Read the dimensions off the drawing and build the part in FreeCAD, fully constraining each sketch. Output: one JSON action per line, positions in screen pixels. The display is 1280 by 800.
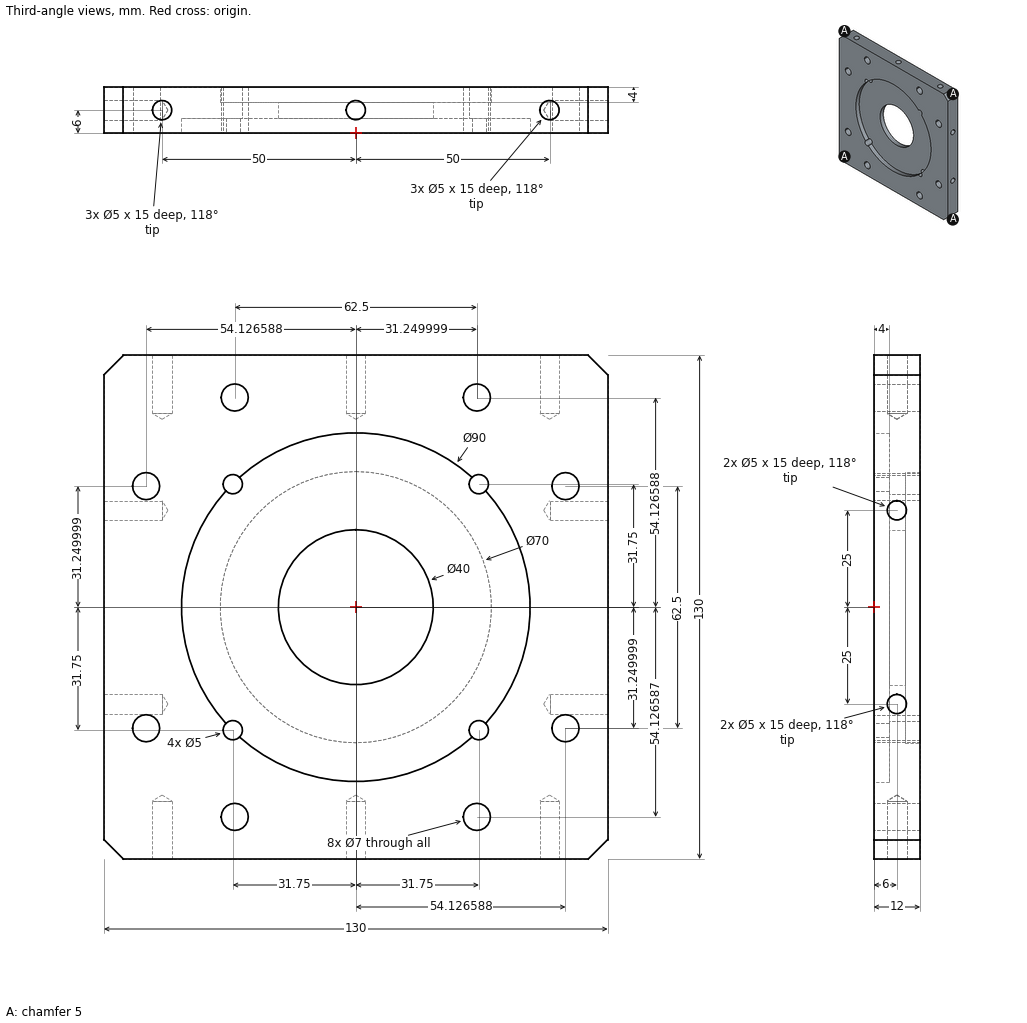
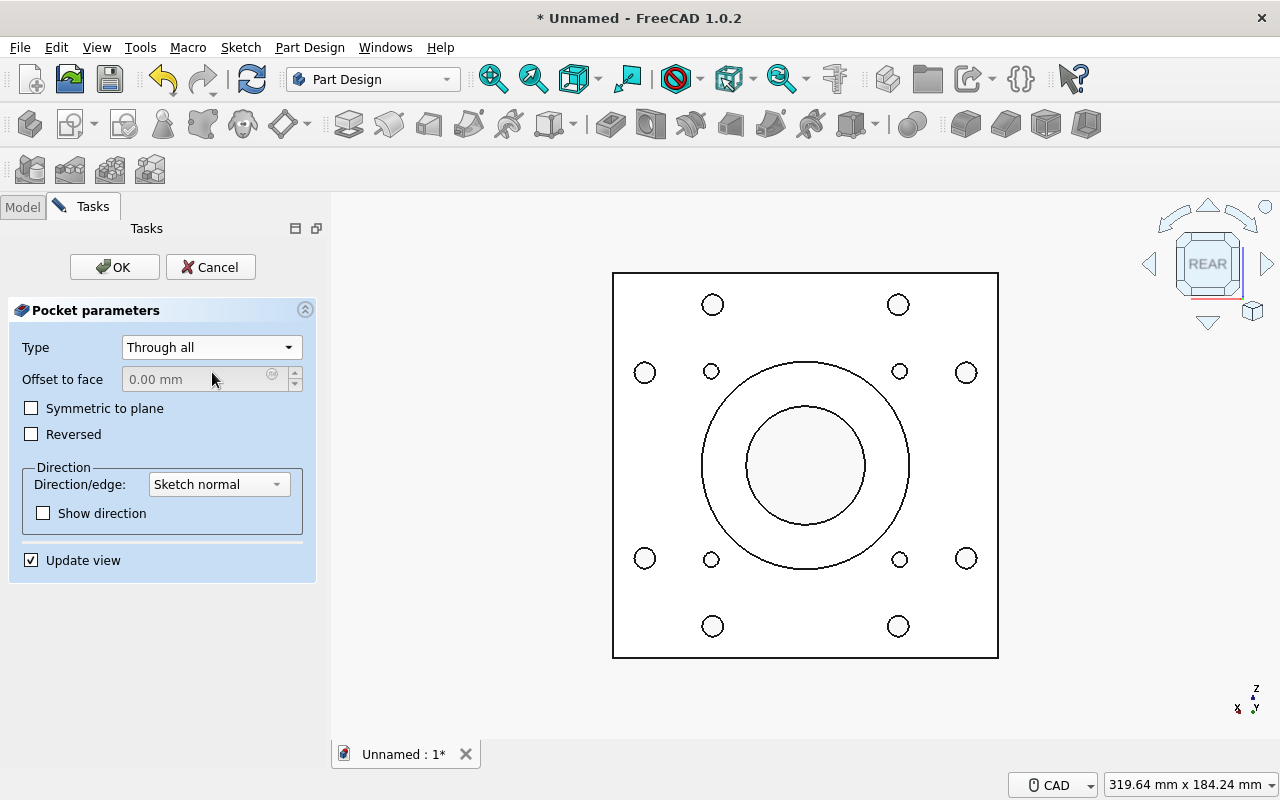
{"action": "left_click", "coordinate": [115, 267]}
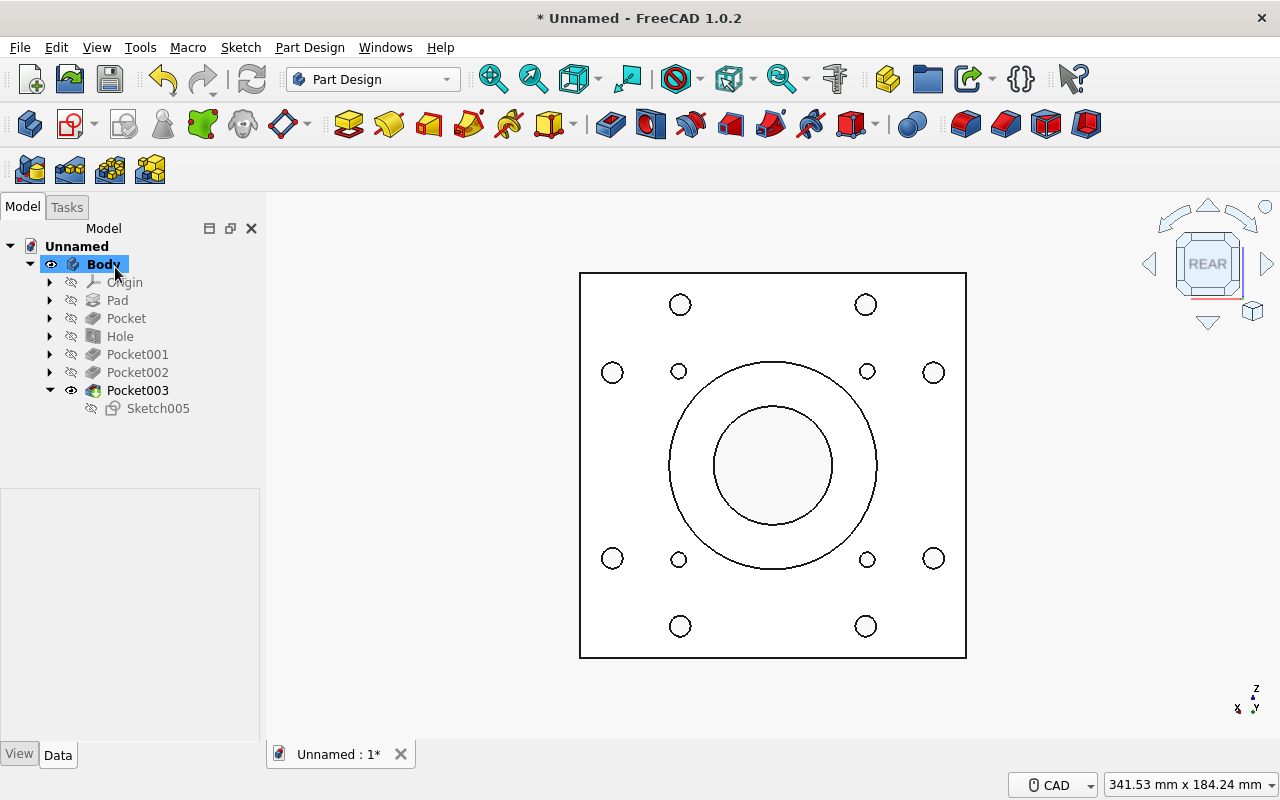
{"action": "key", "text": "6"}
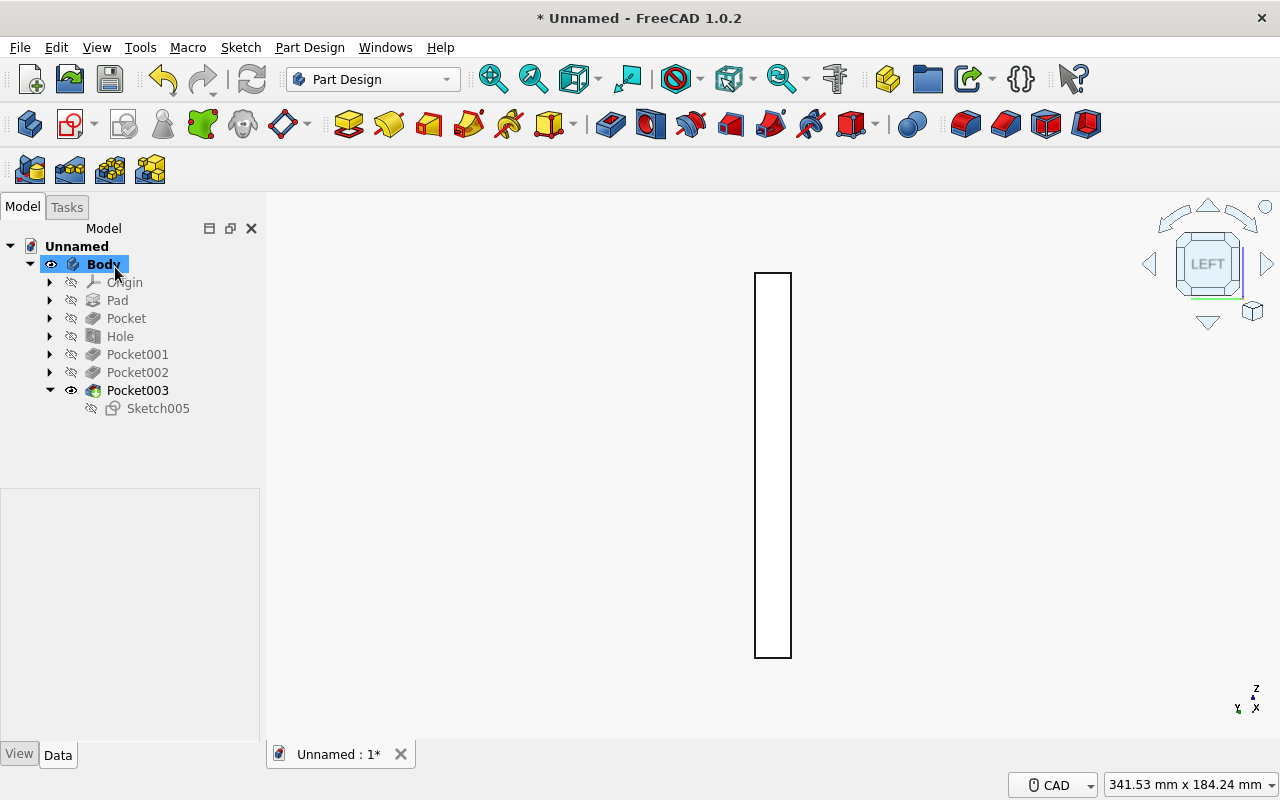
{"action": "left_click", "coordinate": [773, 299]}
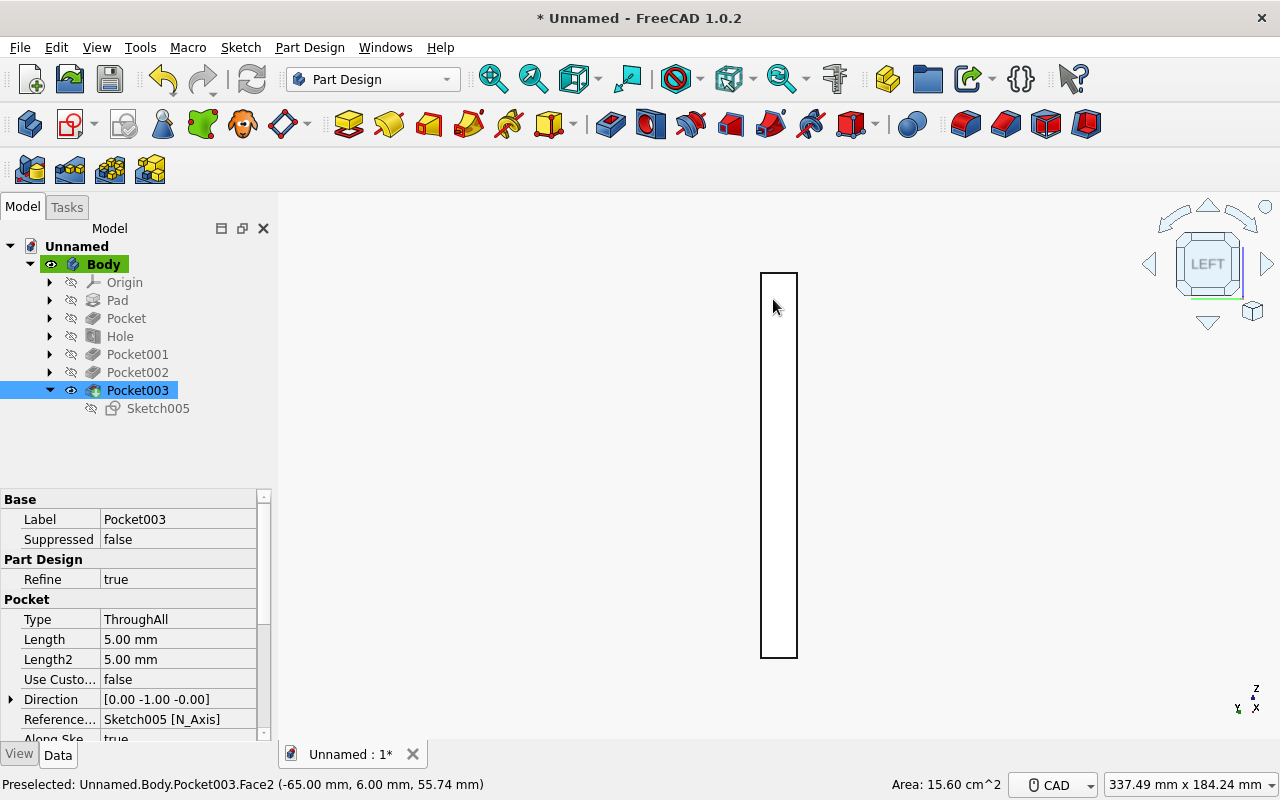
{"action": "left_click", "coordinate": [70, 124]}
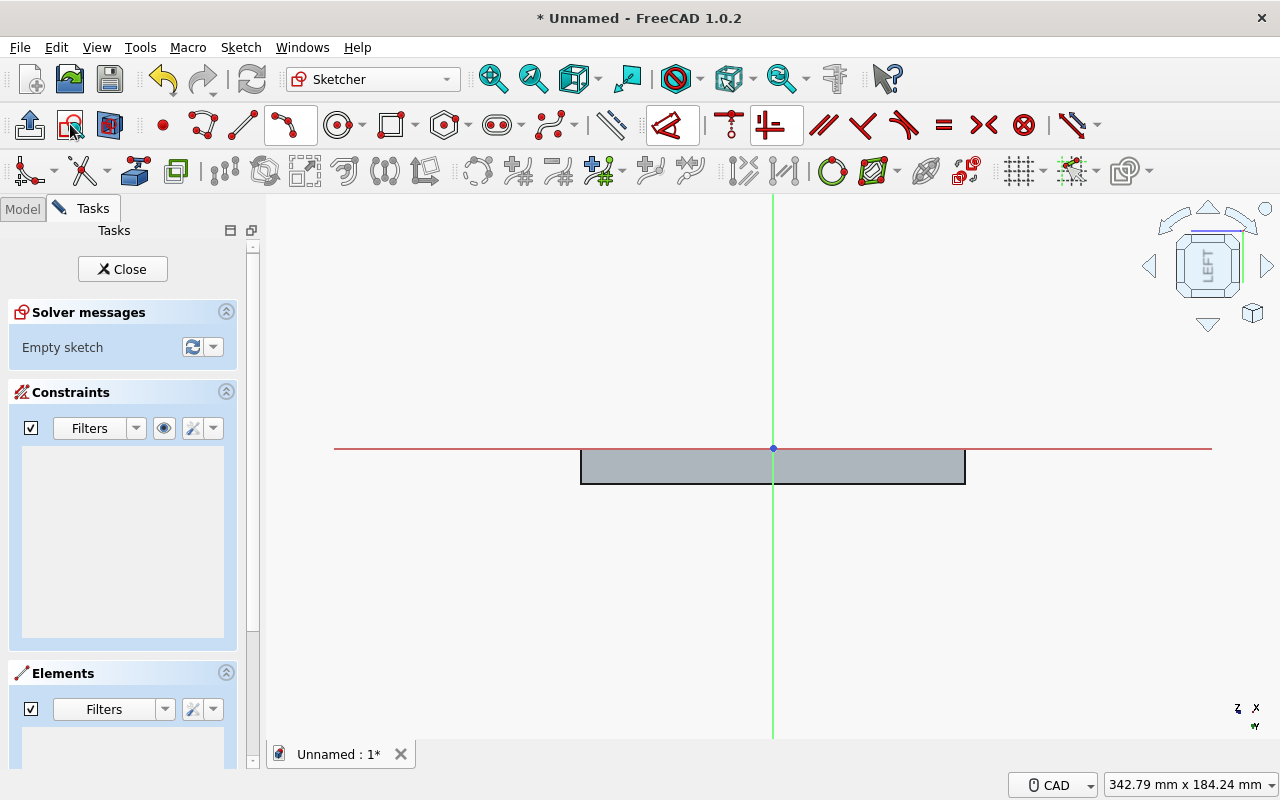
{"action": "scroll", "coordinate": [803, 459], "scroll_direction": "up", "scroll_amount": 6}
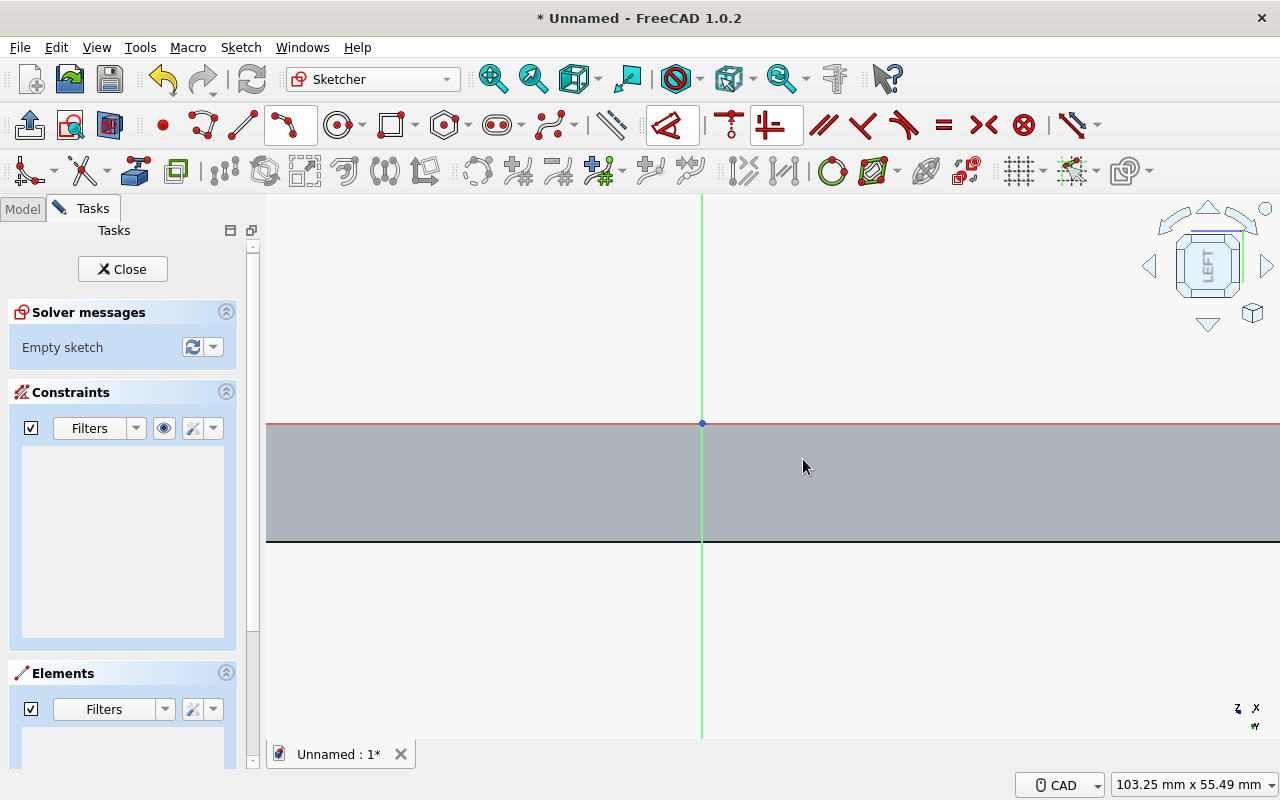
{"action": "left_click", "coordinate": [338, 126]}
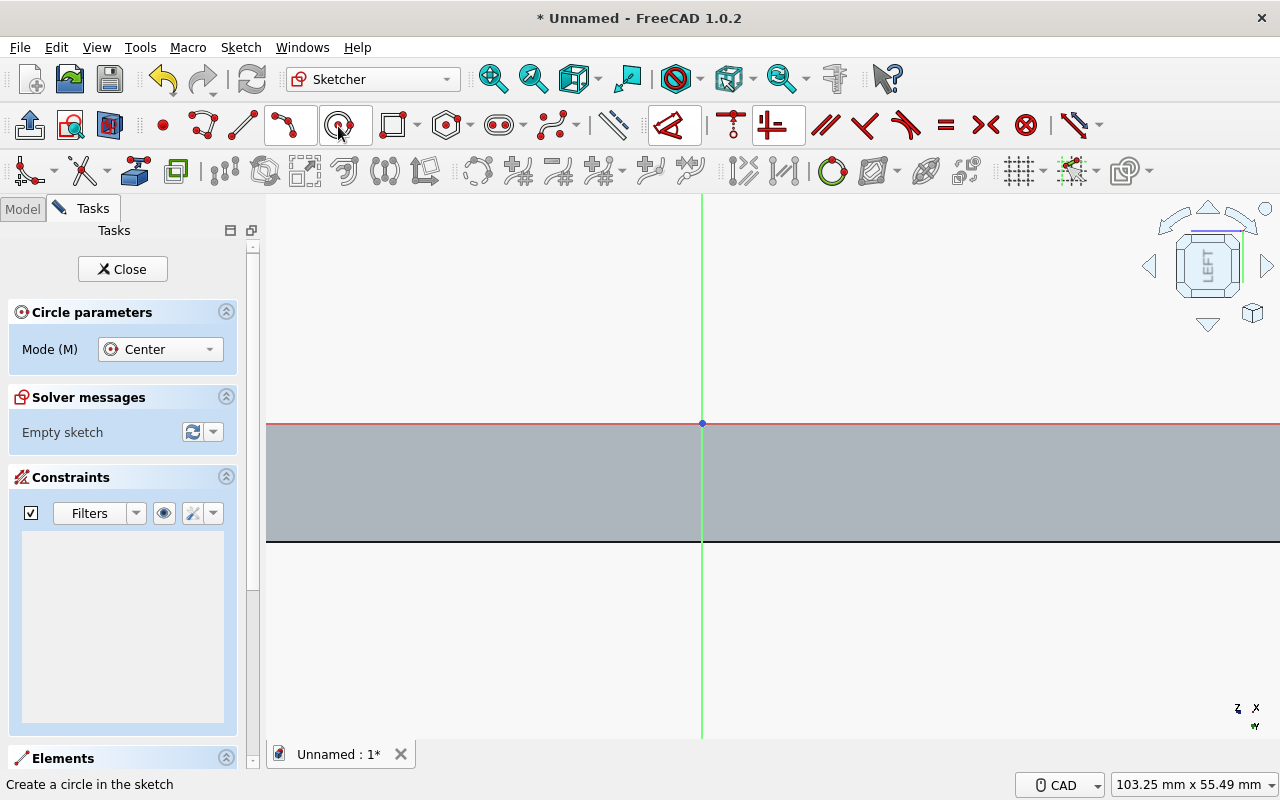
{"action": "left_click", "coordinate": [948, 483]}
{"action": "left_click", "coordinate": [965, 465]}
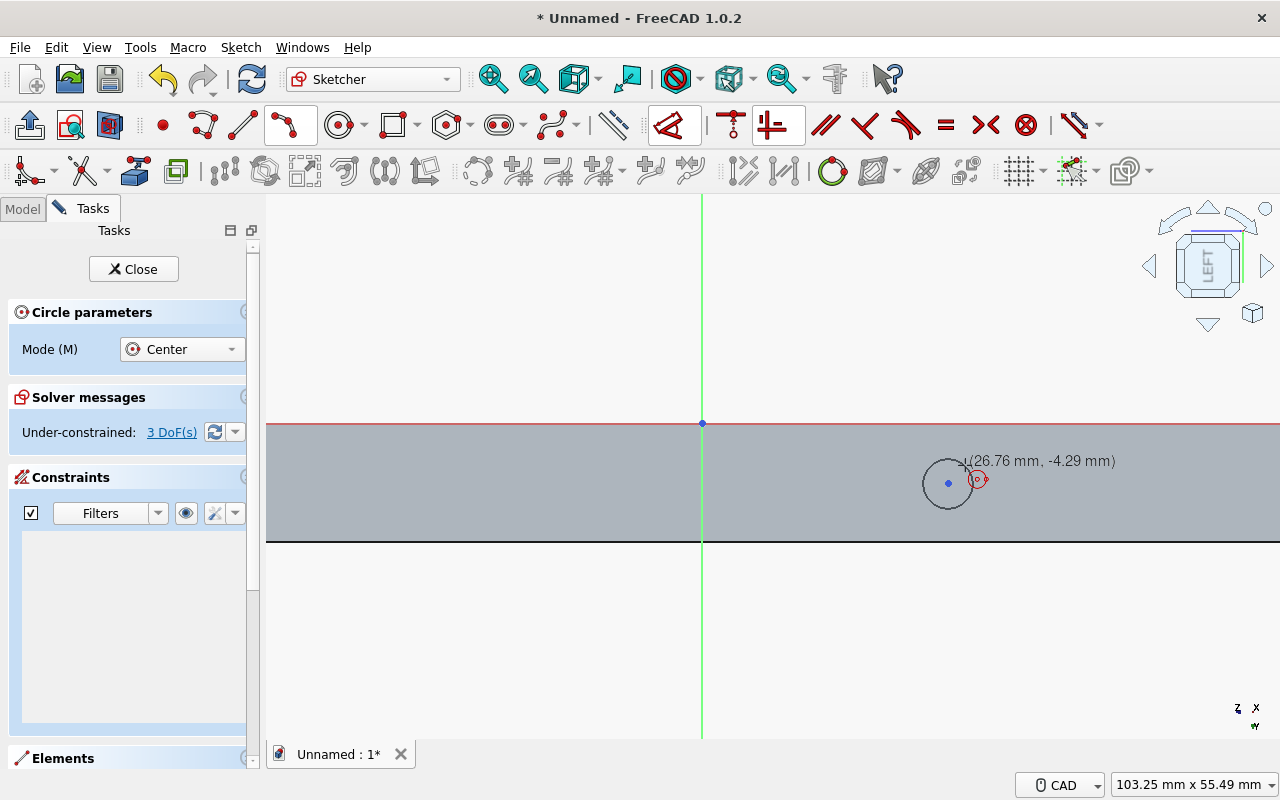
{"action": "left_click", "coordinate": [457, 483]}
{"action": "left_click", "coordinate": [474, 465]}
{"action": "key", "text": "Escape"}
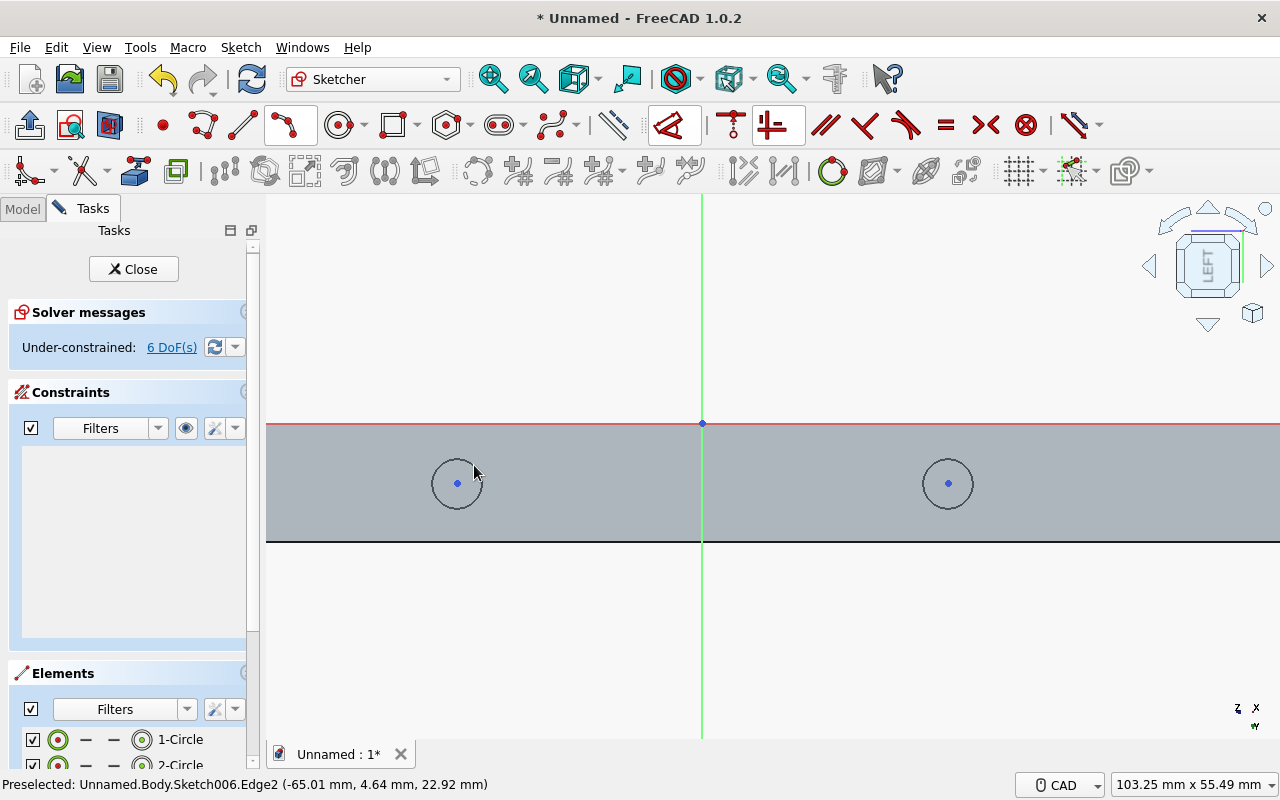
{"action": "left_click", "coordinate": [965, 466]}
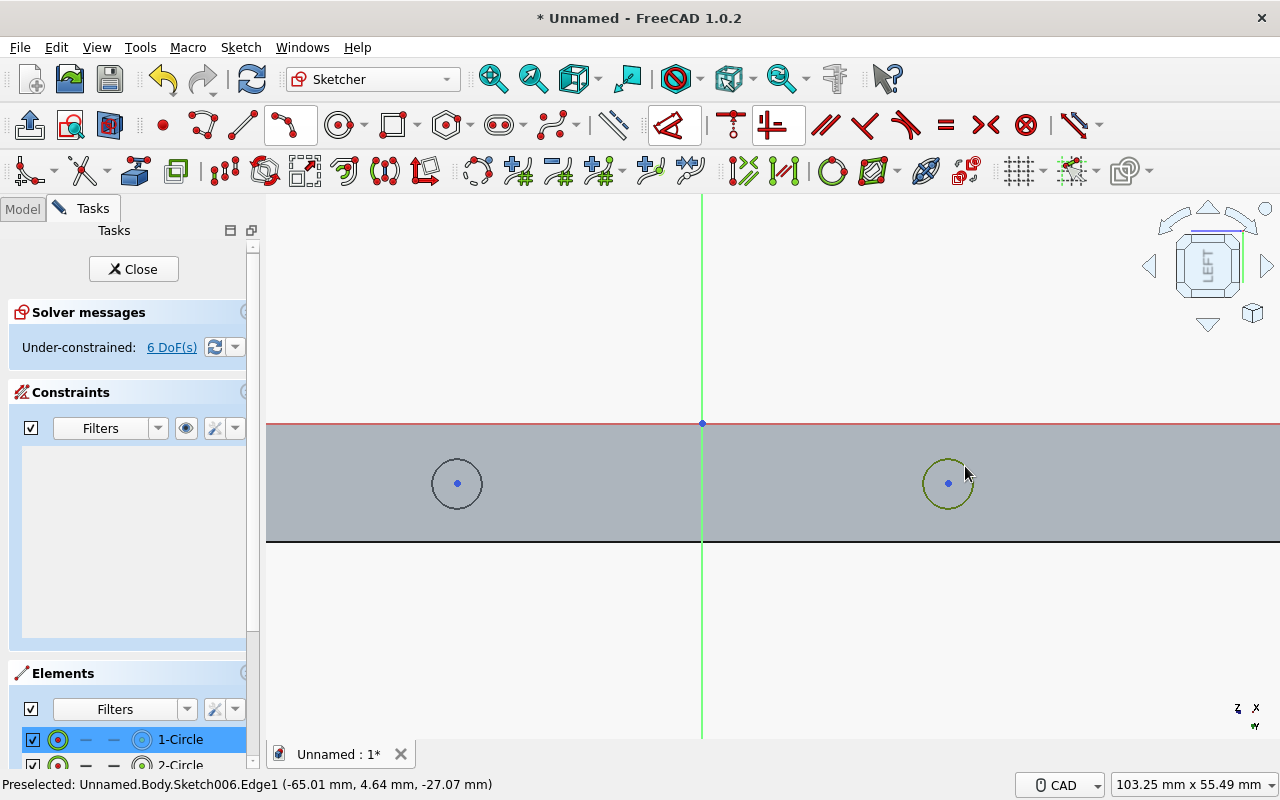
{"action": "left_click", "coordinate": [474, 466]}